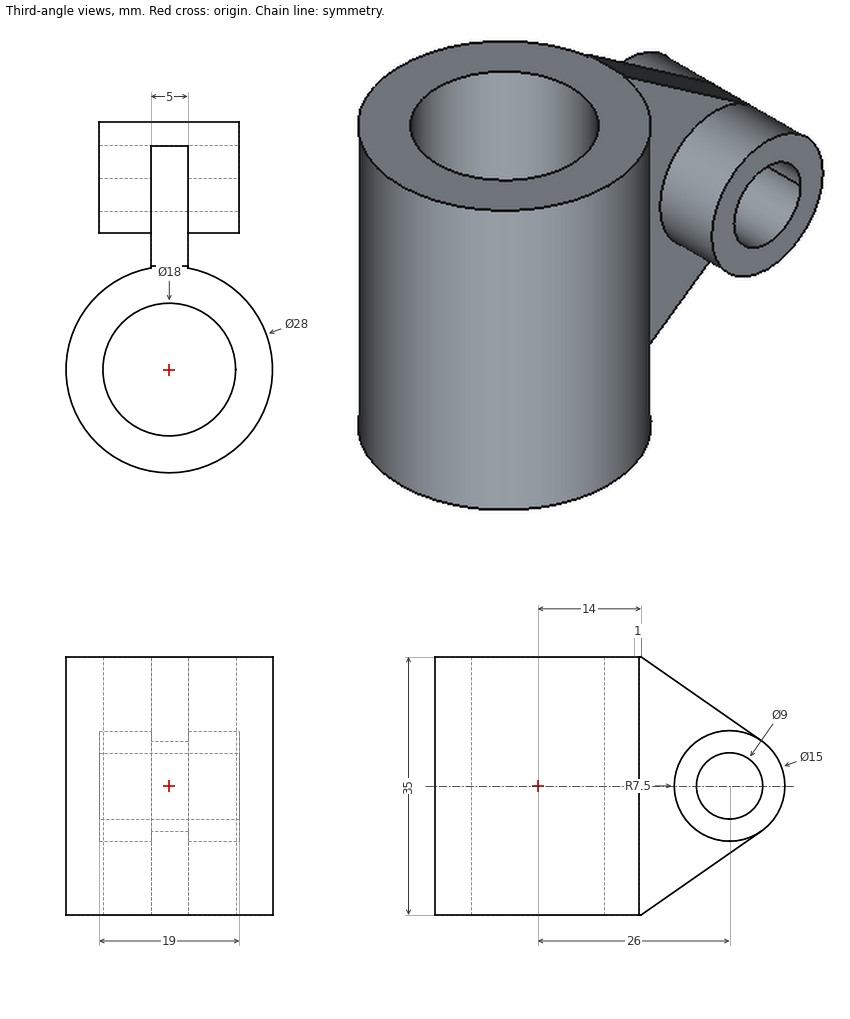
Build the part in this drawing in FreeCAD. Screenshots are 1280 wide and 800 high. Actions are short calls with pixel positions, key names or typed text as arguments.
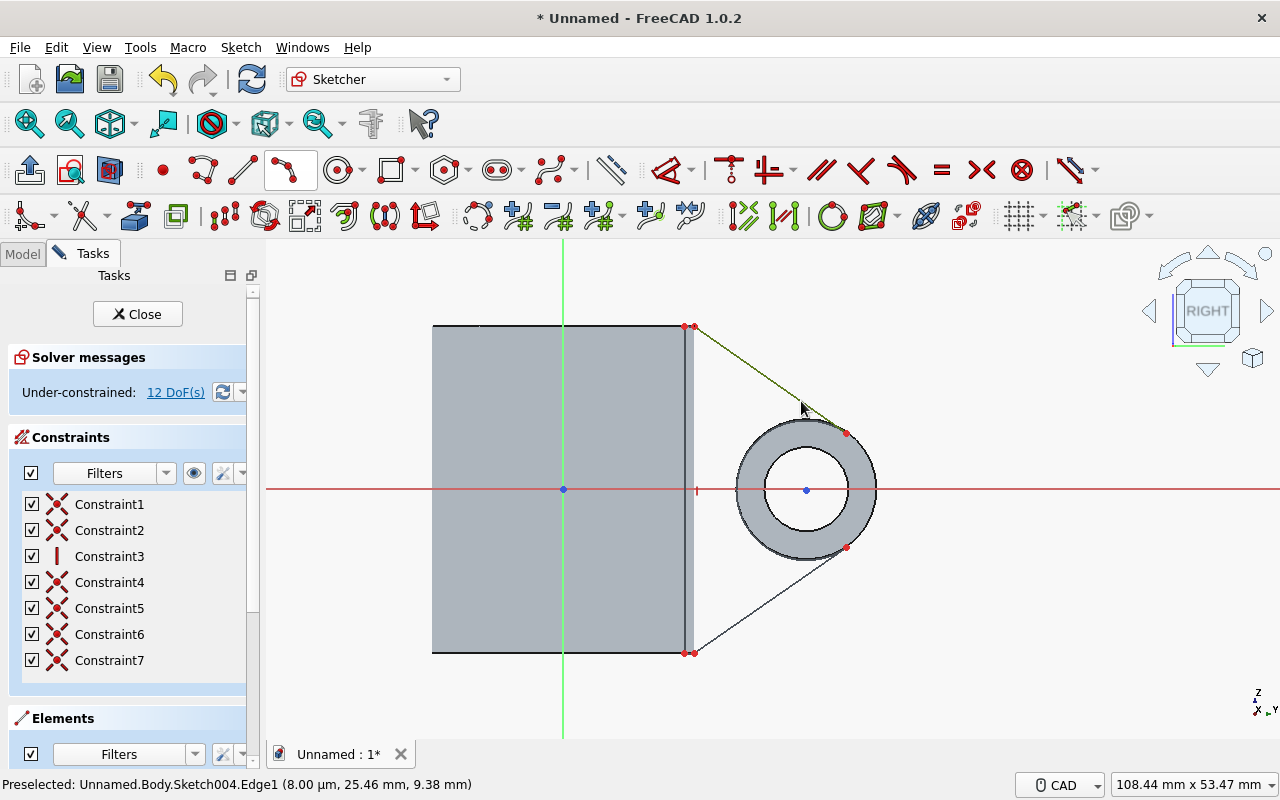
click(761, 437)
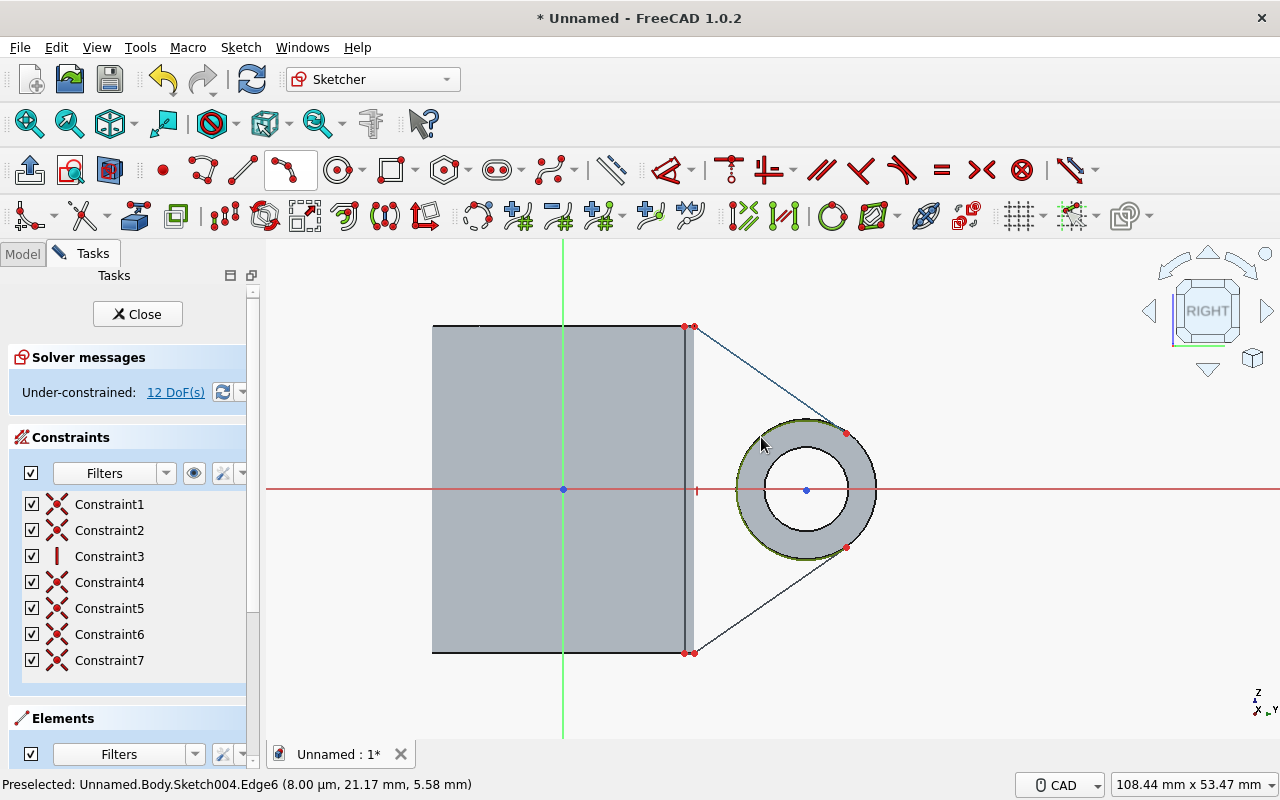
click(902, 170)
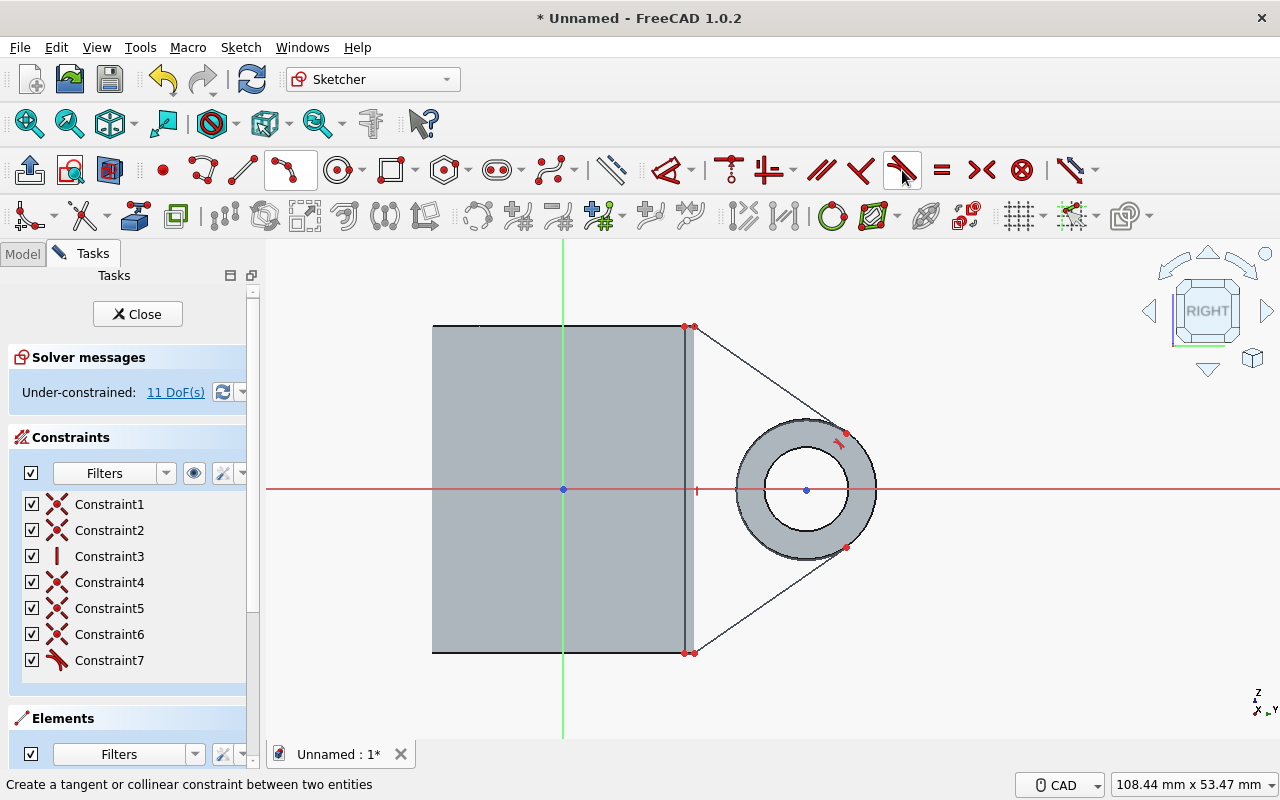
click(740, 622)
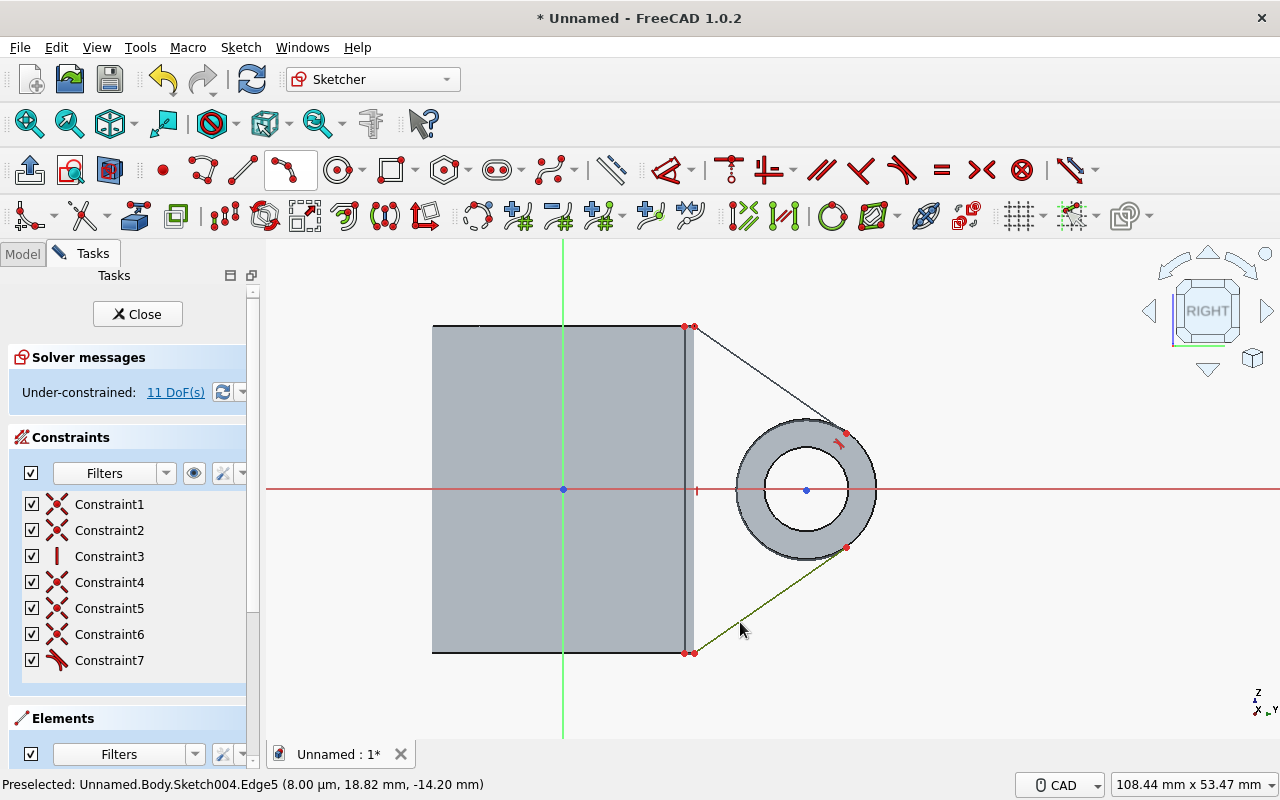
click(761, 437)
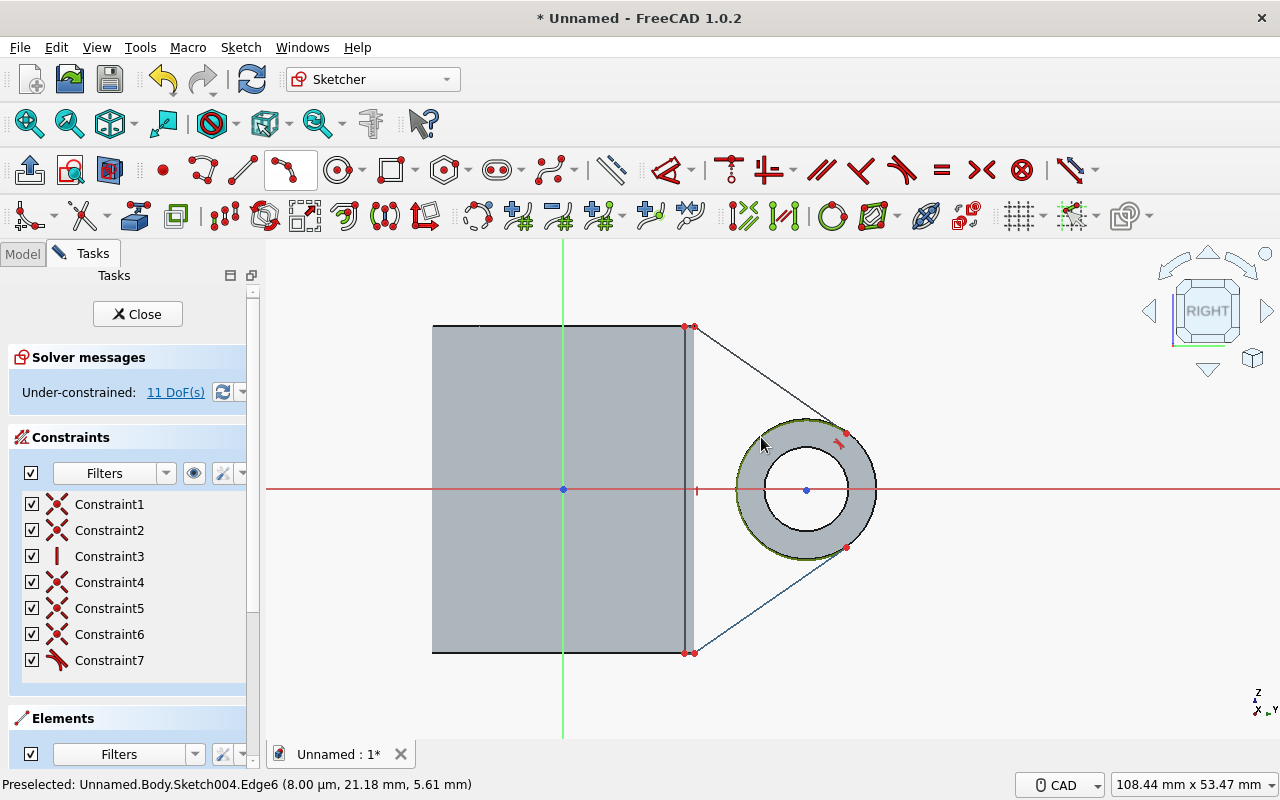
key(t)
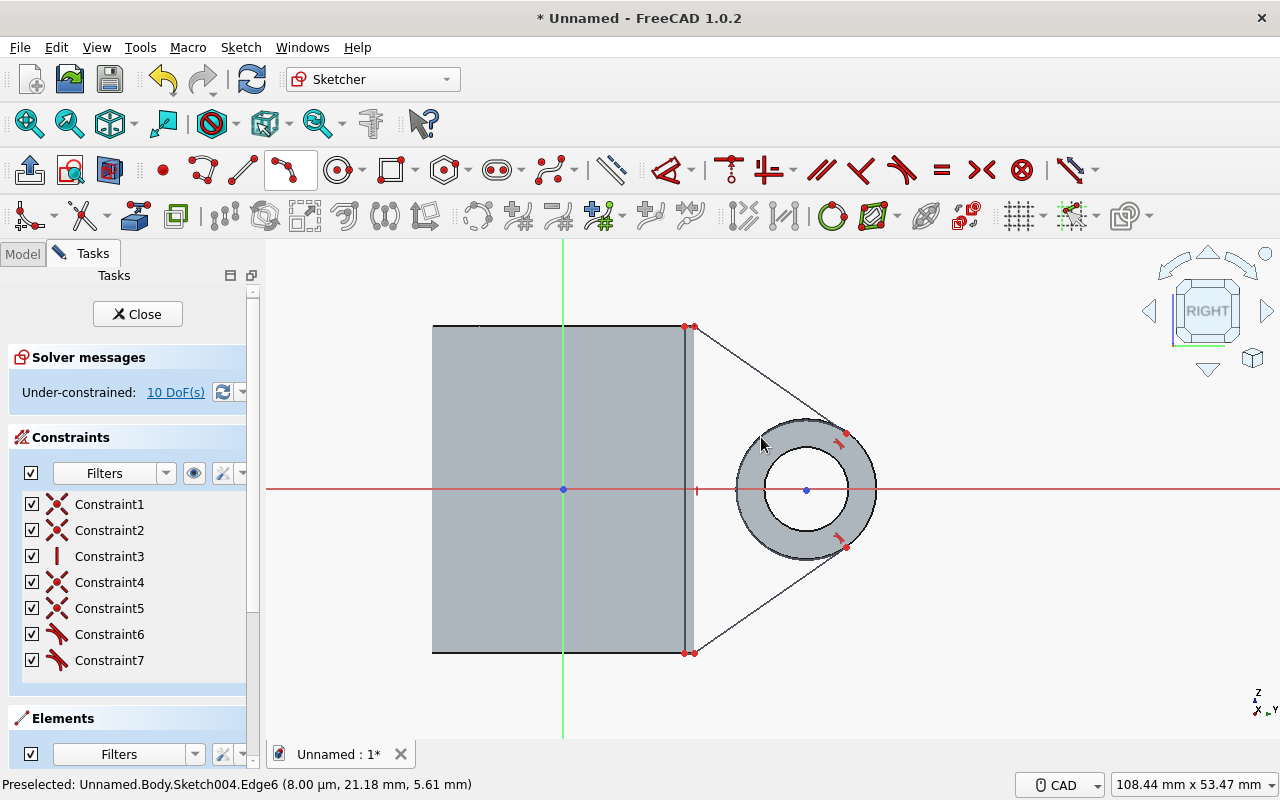
scroll(690, 327, up, 6)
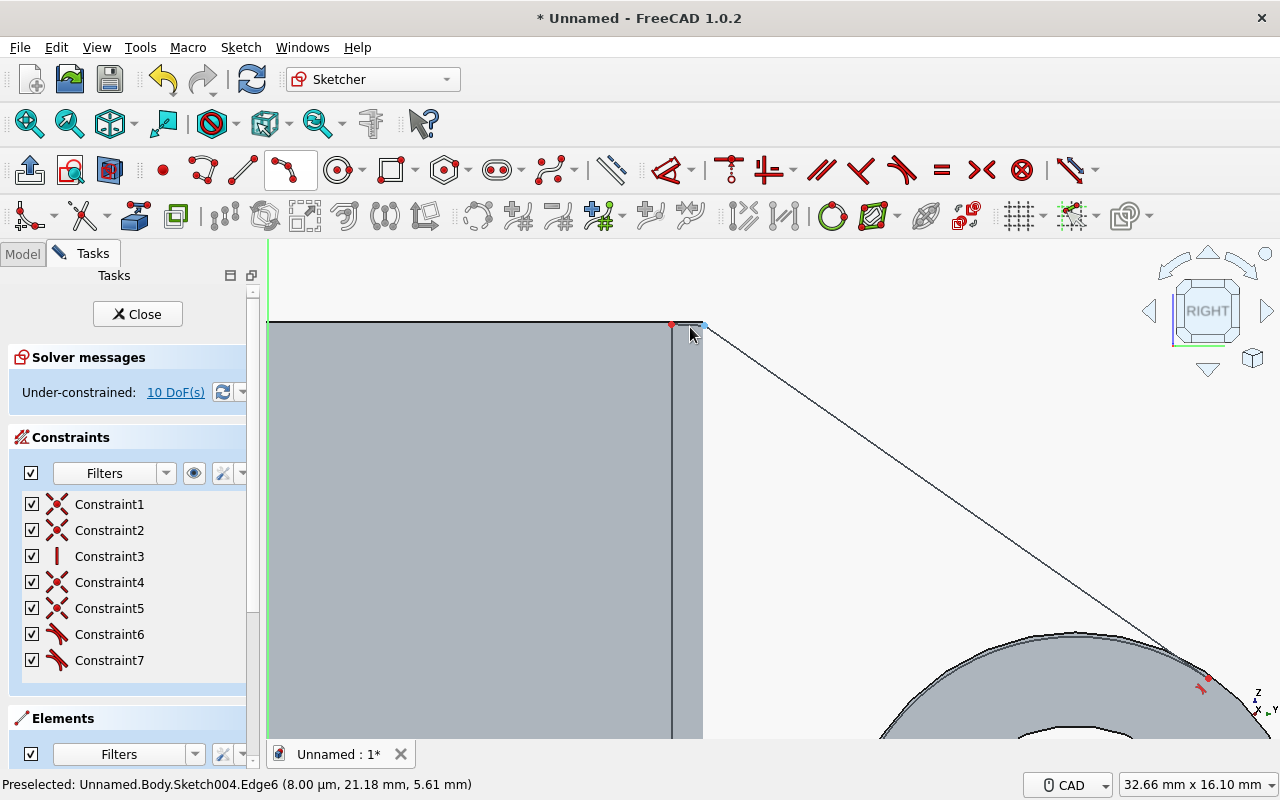
click(688, 325)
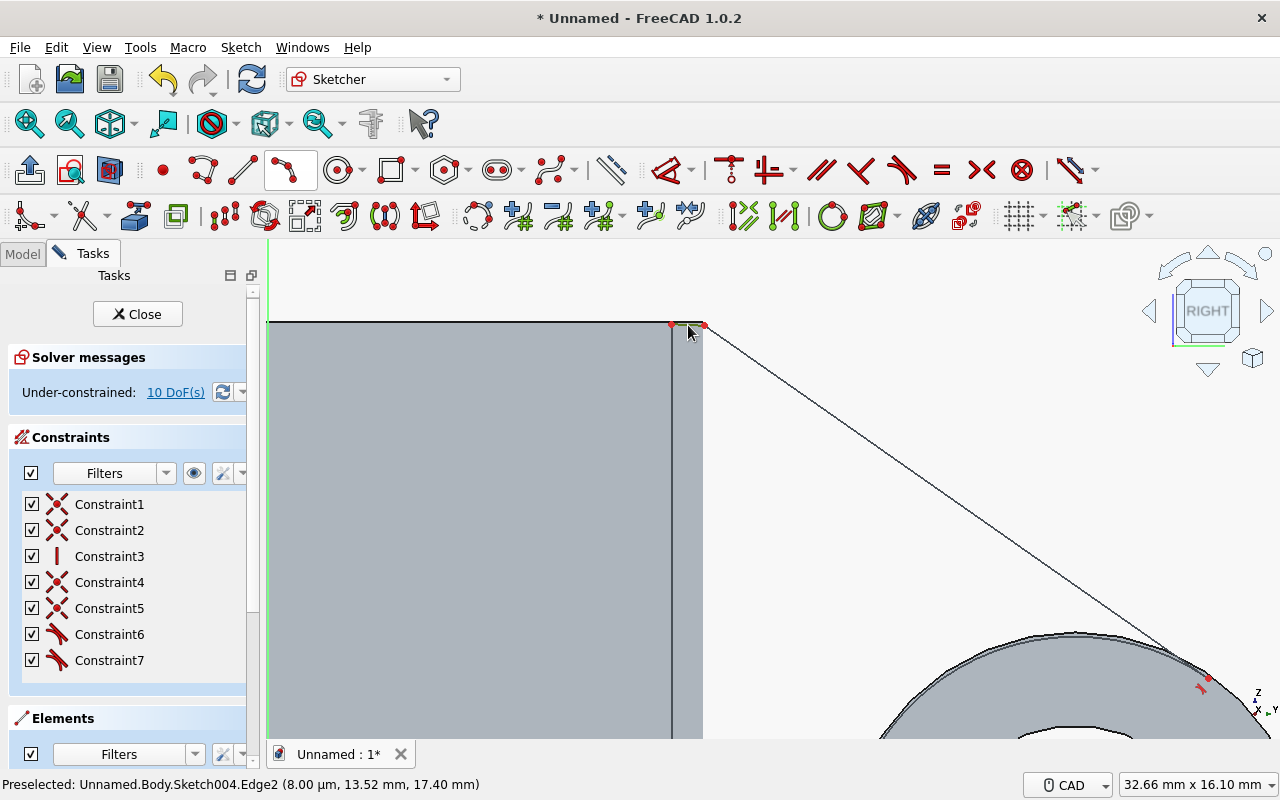
key(h)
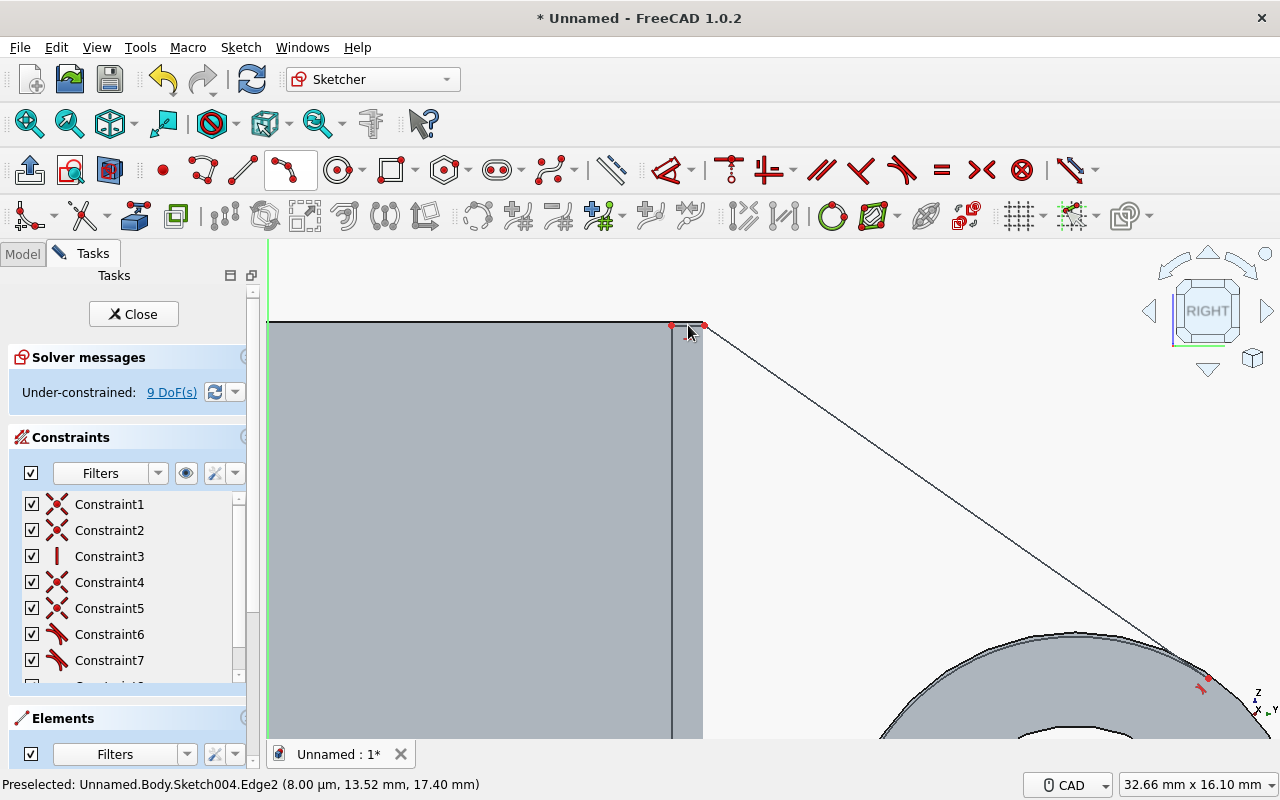
scroll(690, 327, down, 6)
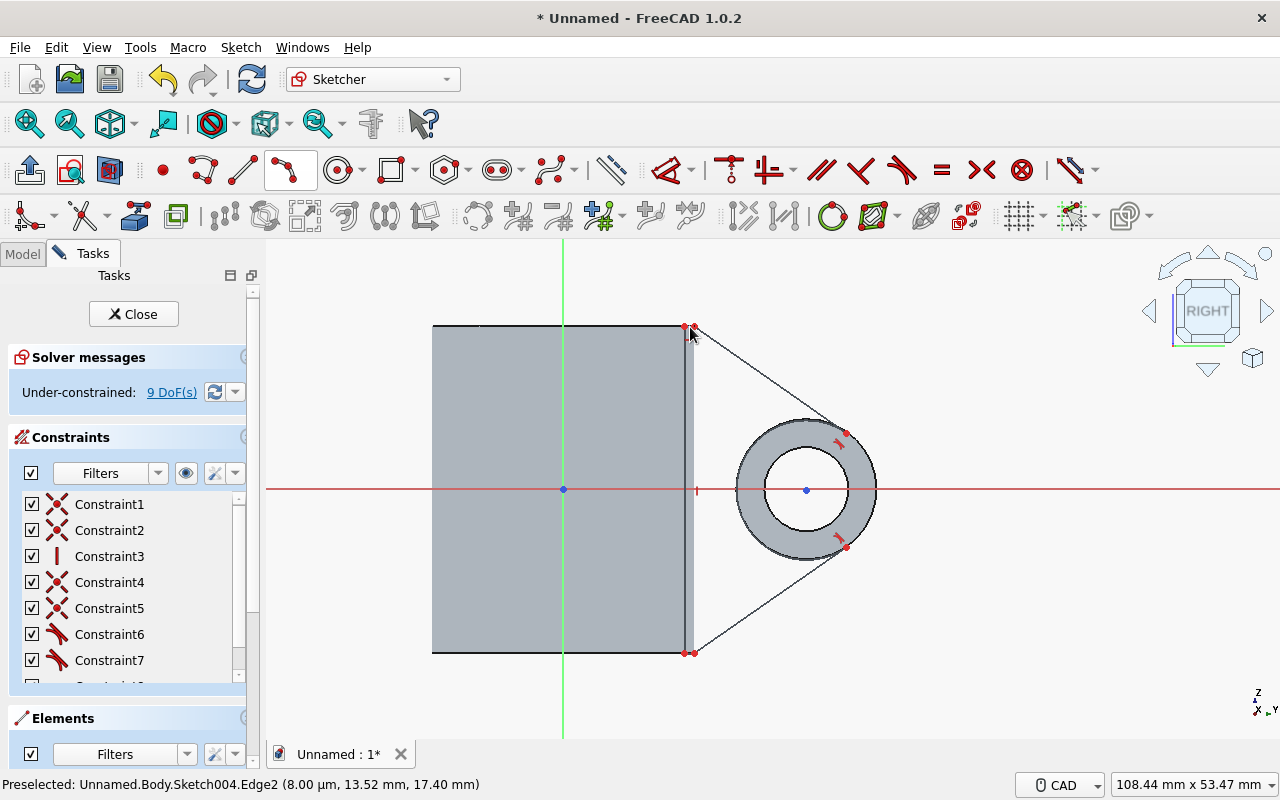
scroll(688, 654, up, 8)